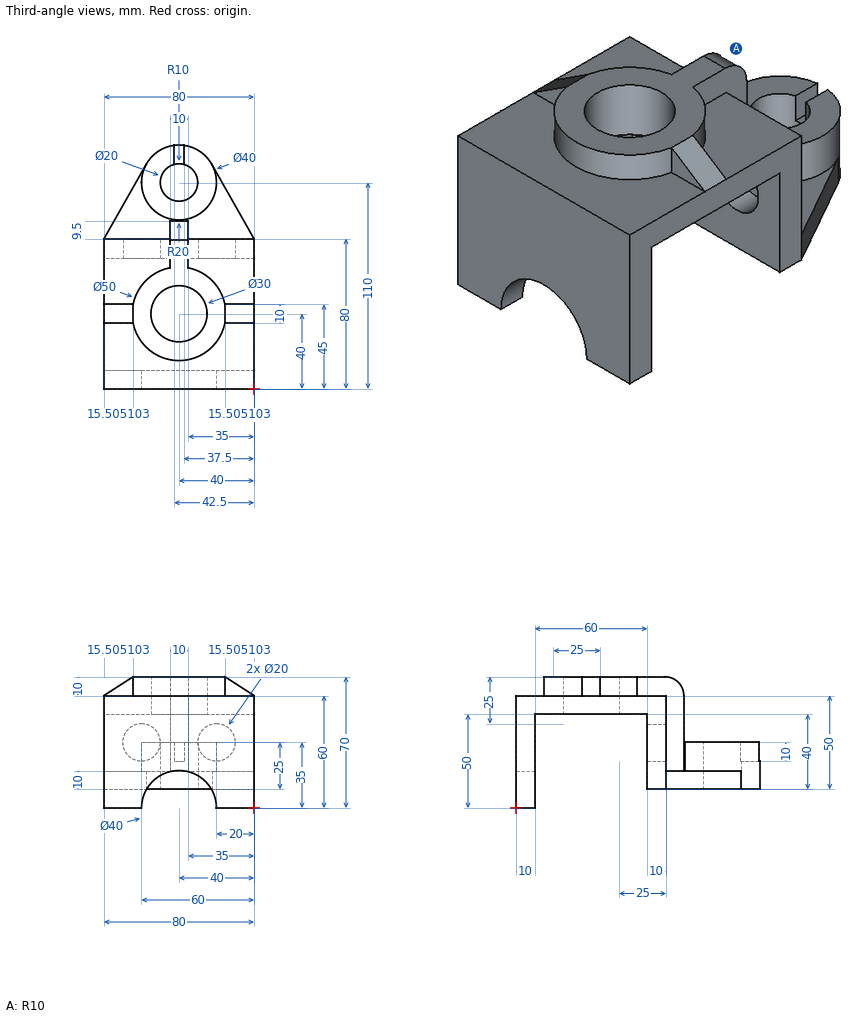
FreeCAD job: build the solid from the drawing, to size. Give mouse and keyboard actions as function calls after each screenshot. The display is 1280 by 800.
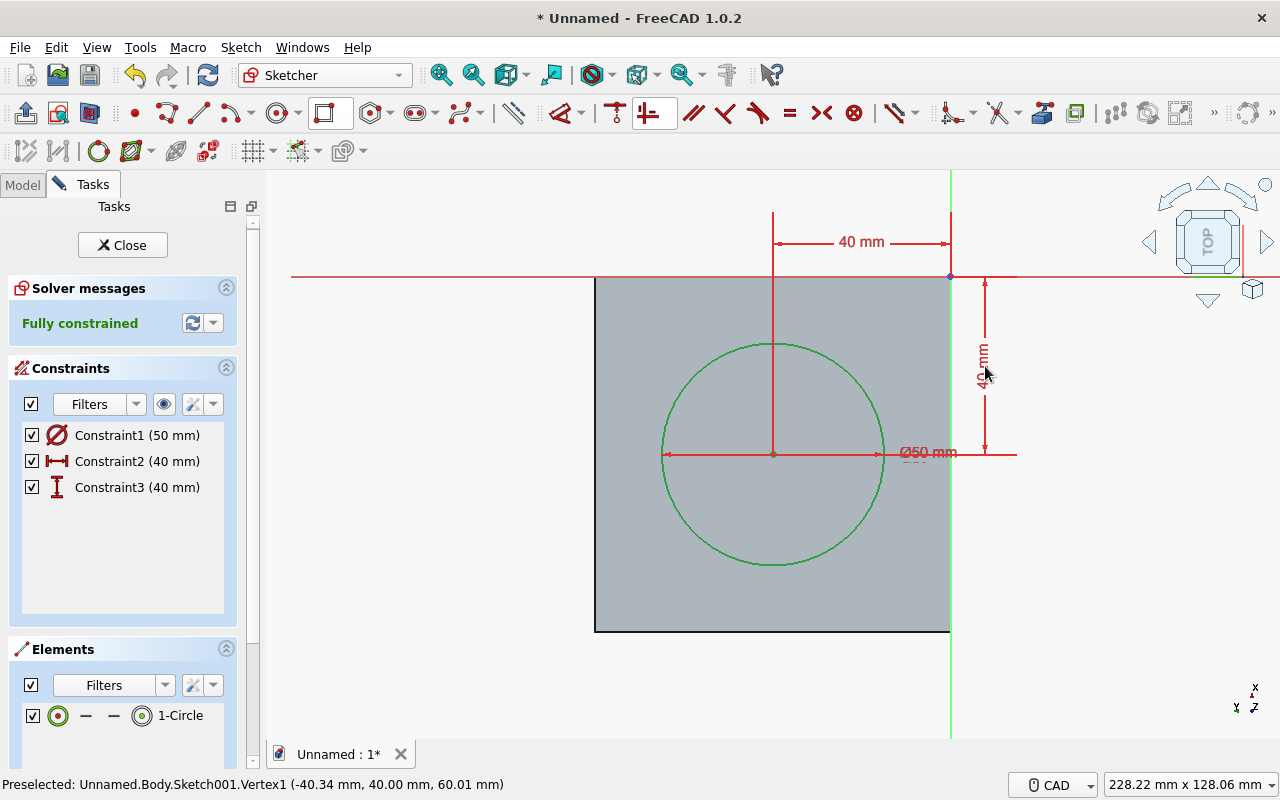
click(123, 245)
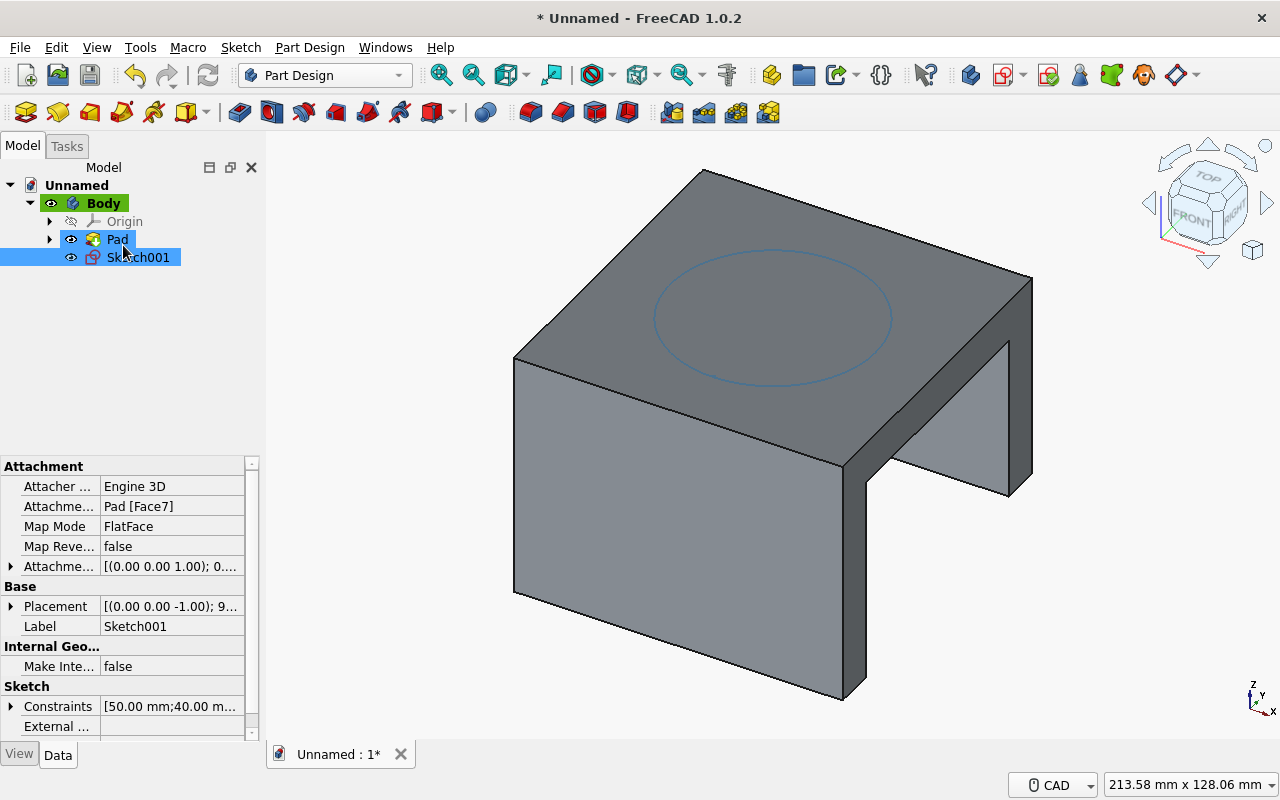
click(26, 112)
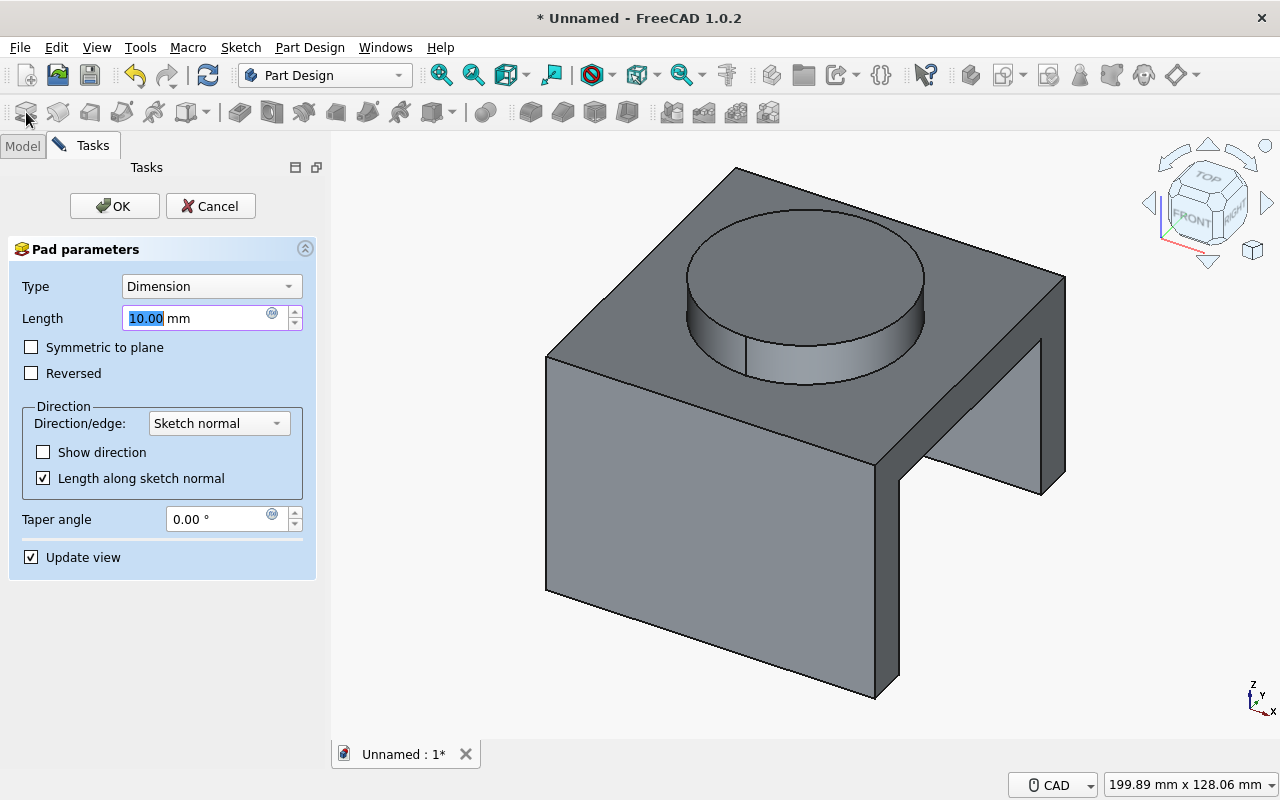
text(10)
key(Tab)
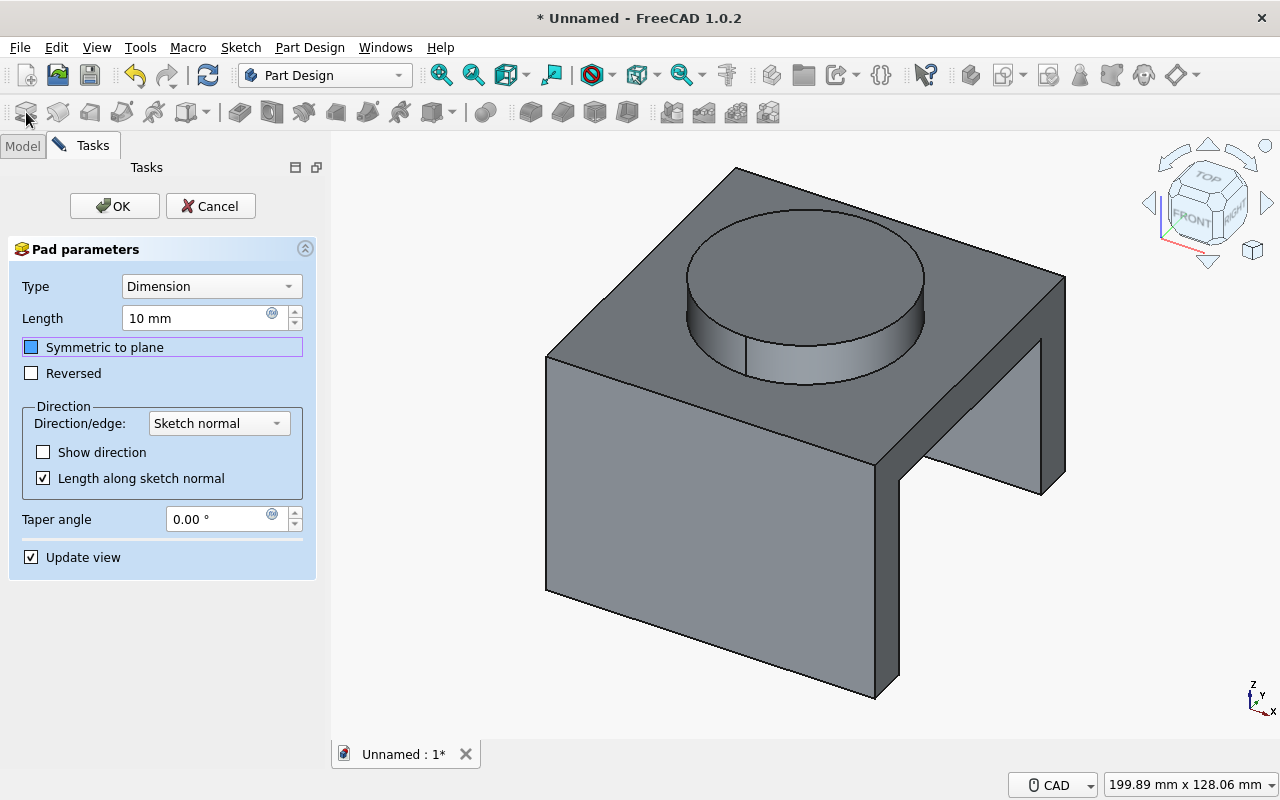
click(115, 206)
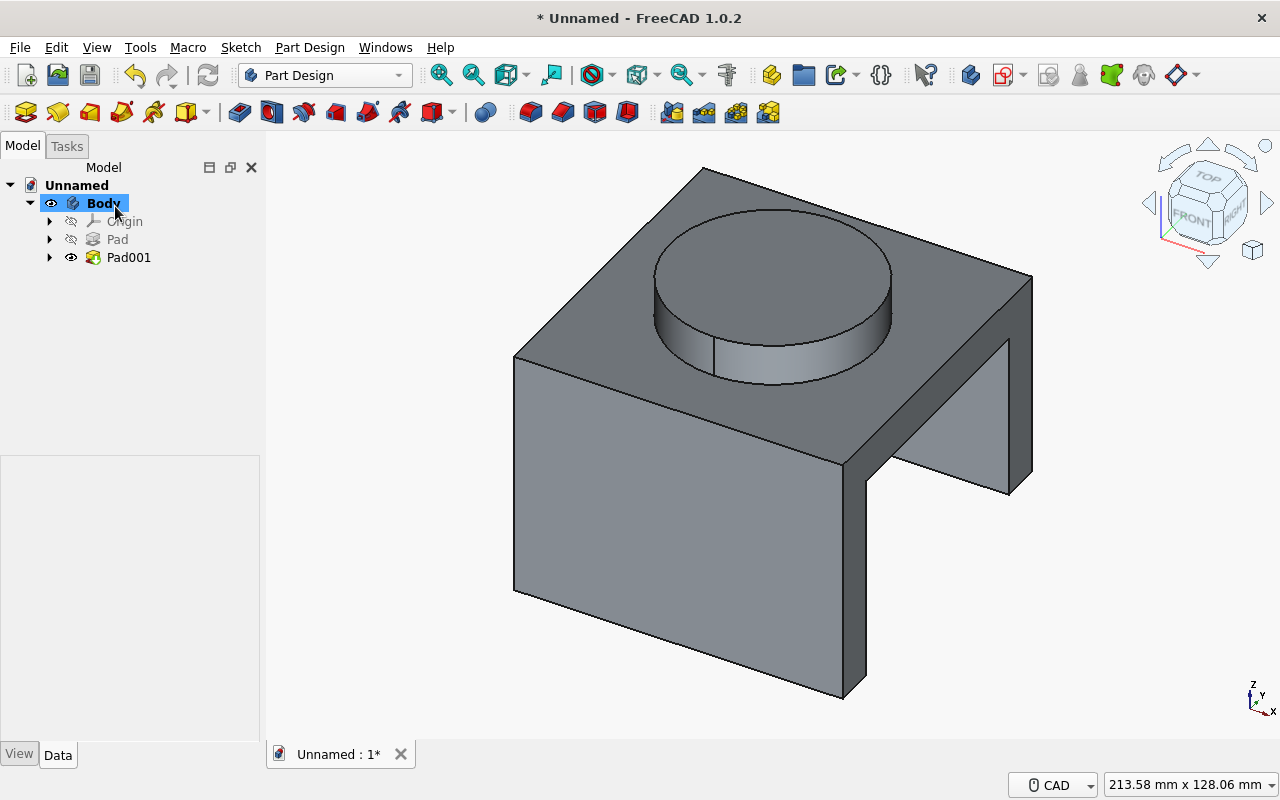
click(442, 76)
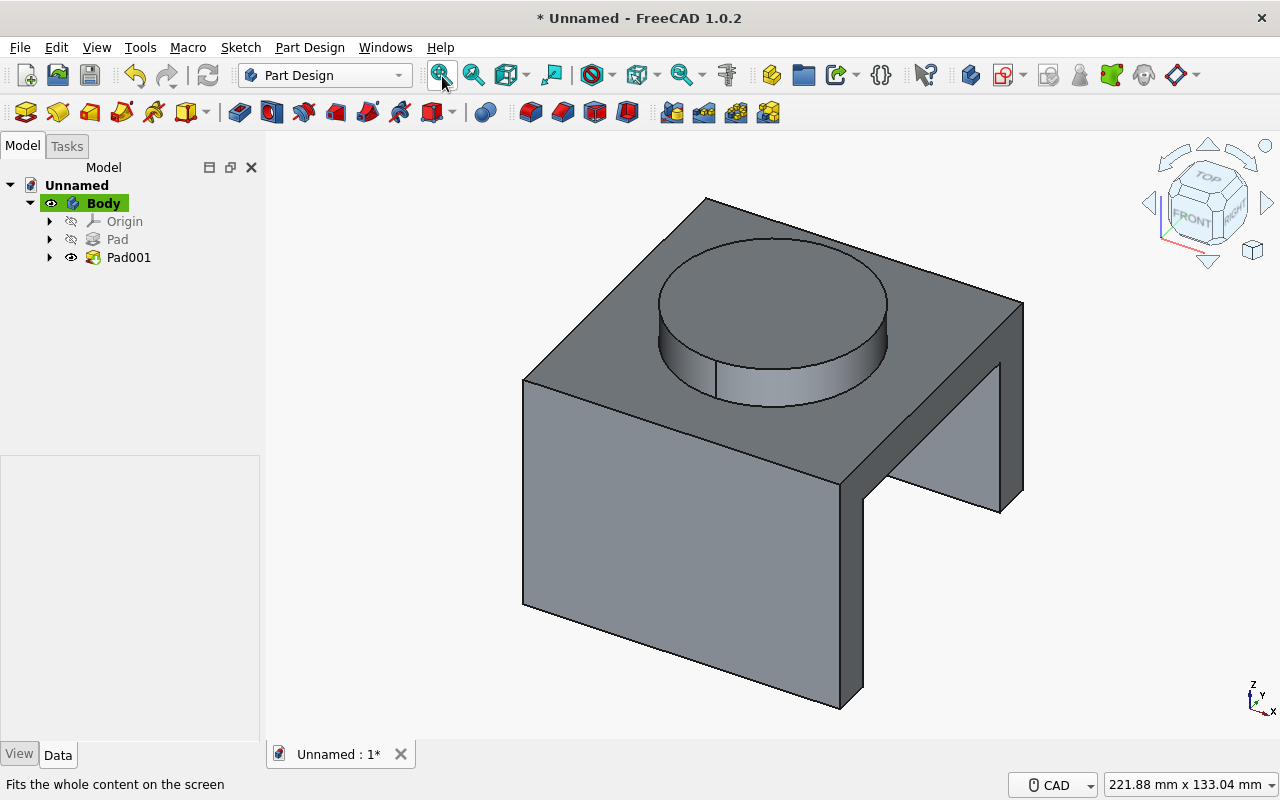
key(5)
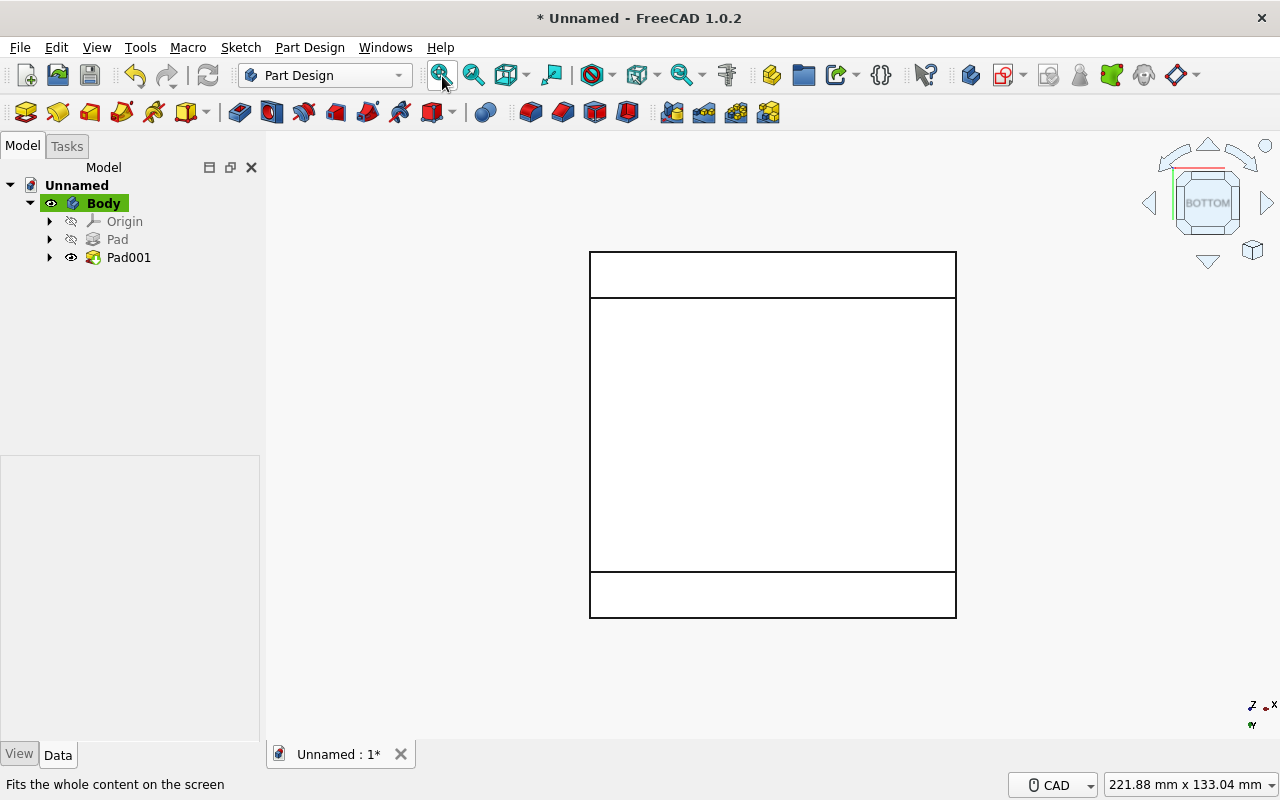
click(877, 594)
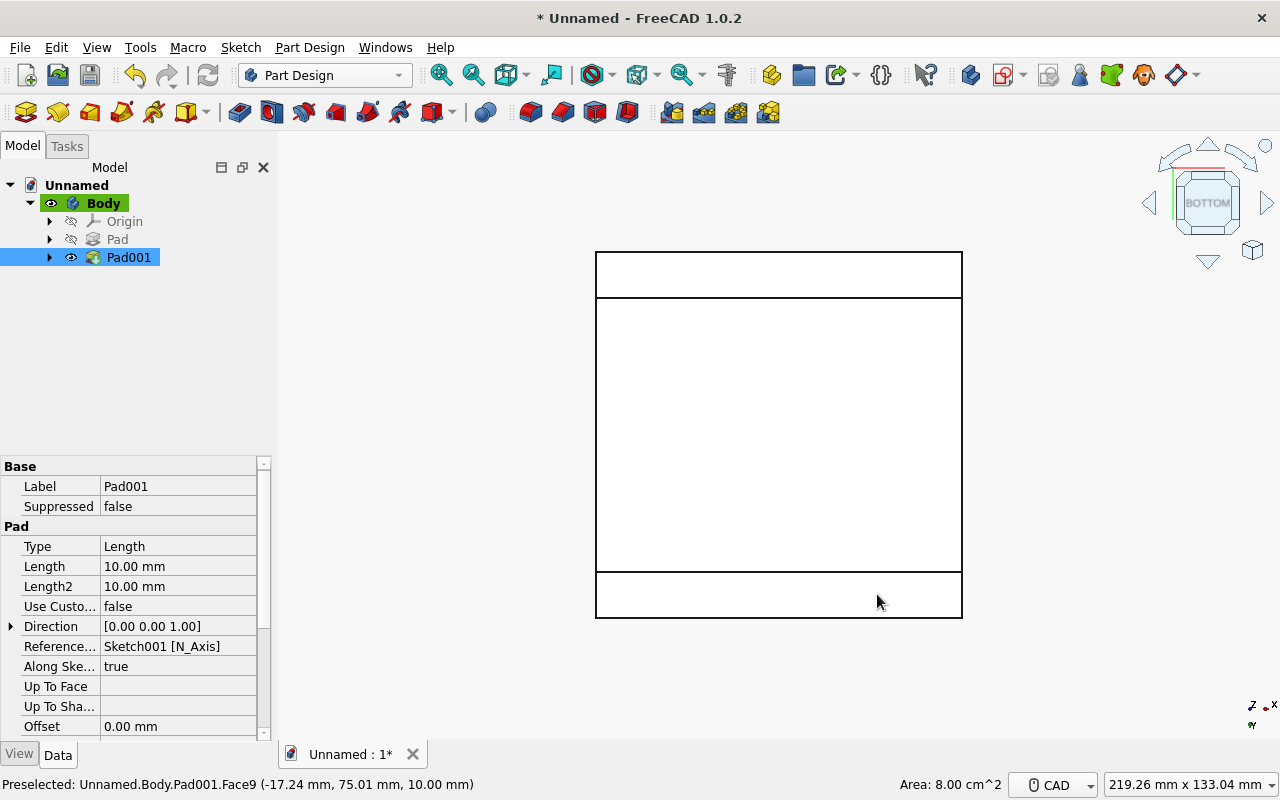
click(1004, 76)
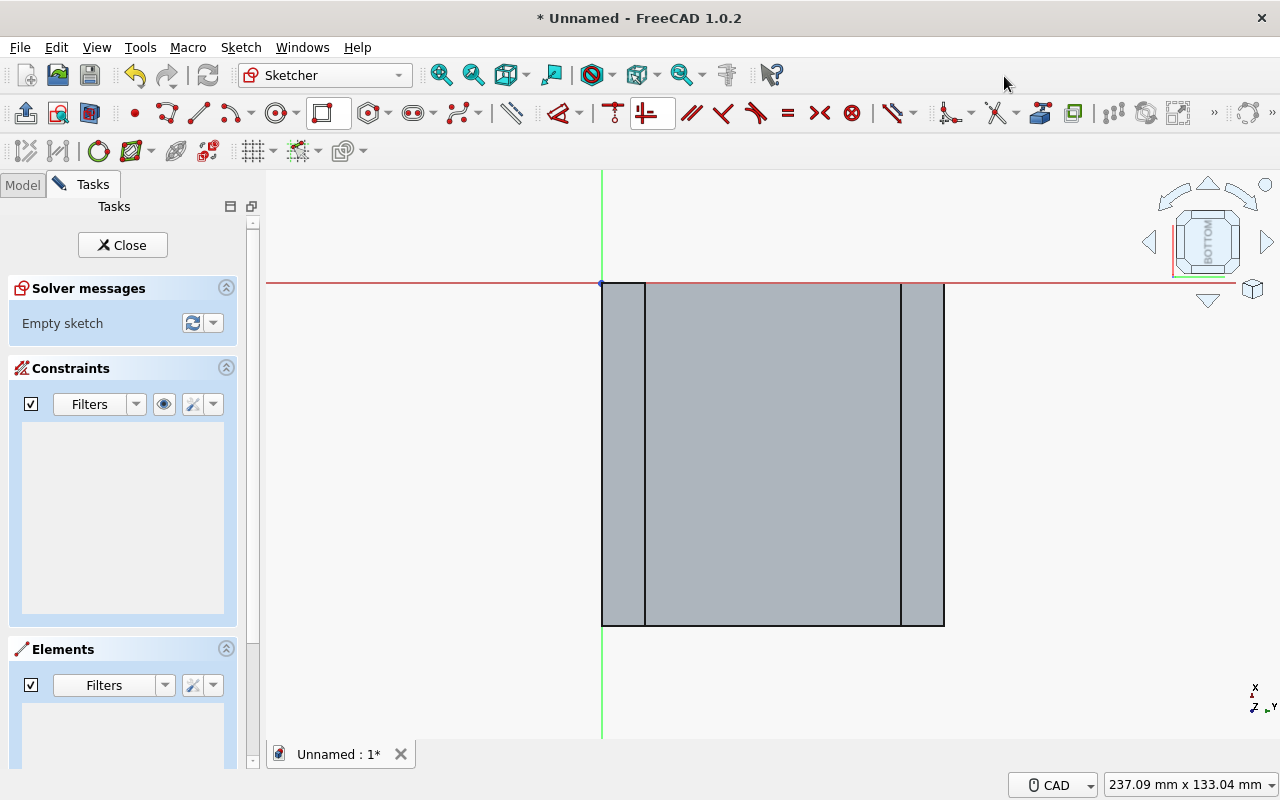
scroll(294, 455, down, 1)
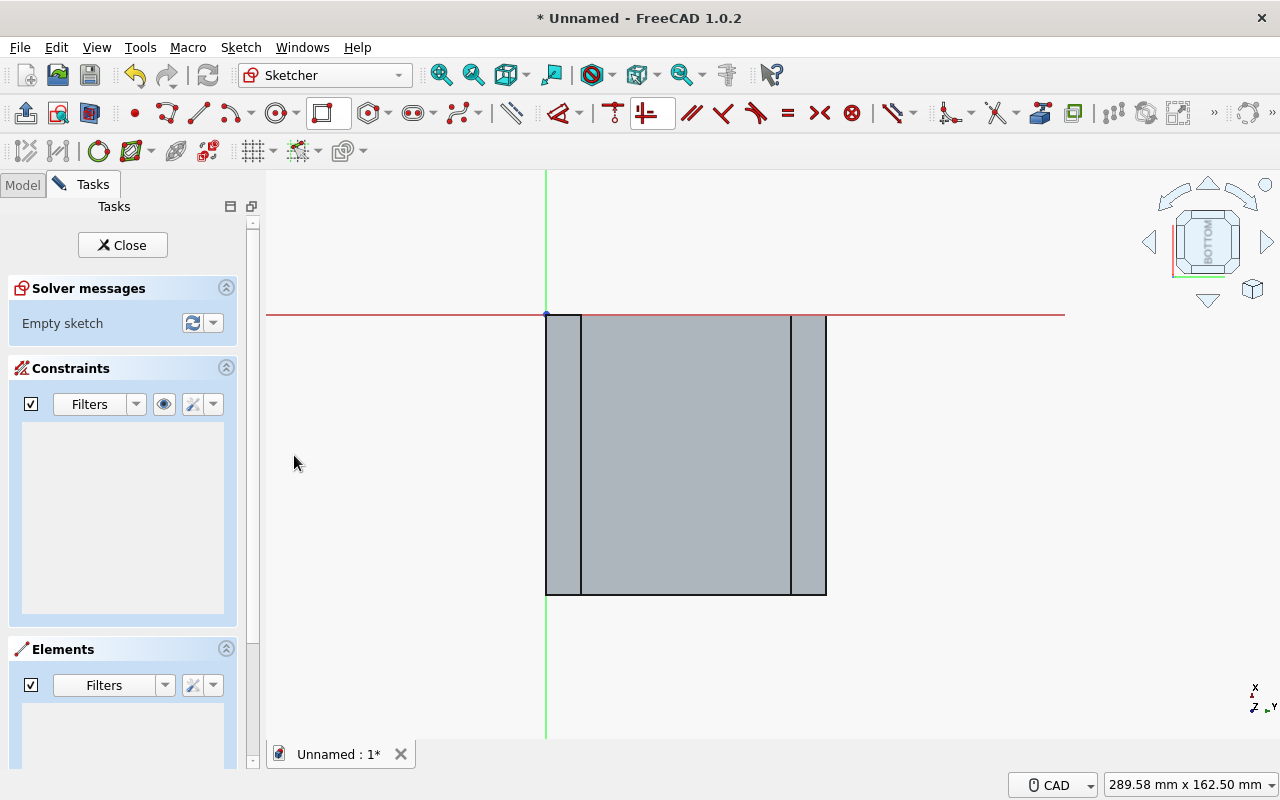
click(168, 114)